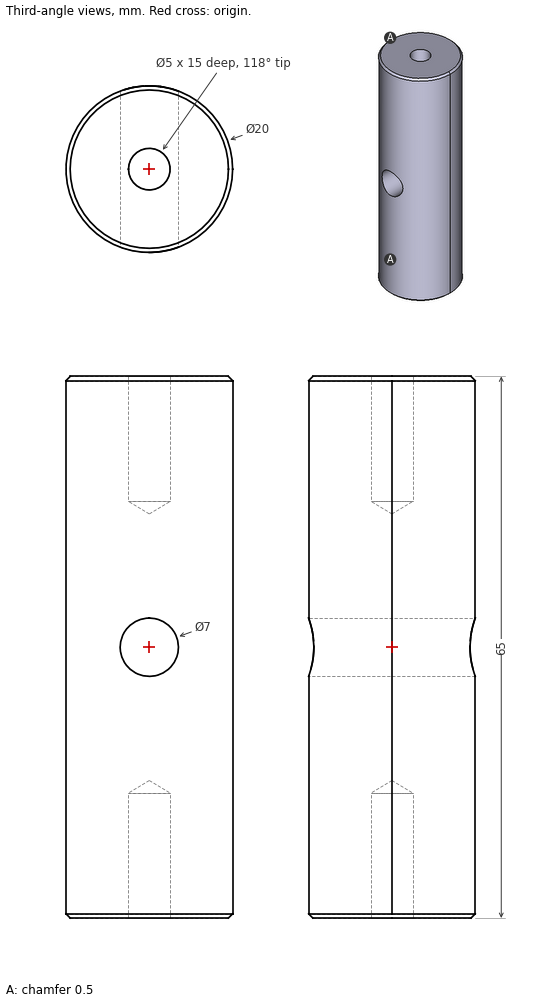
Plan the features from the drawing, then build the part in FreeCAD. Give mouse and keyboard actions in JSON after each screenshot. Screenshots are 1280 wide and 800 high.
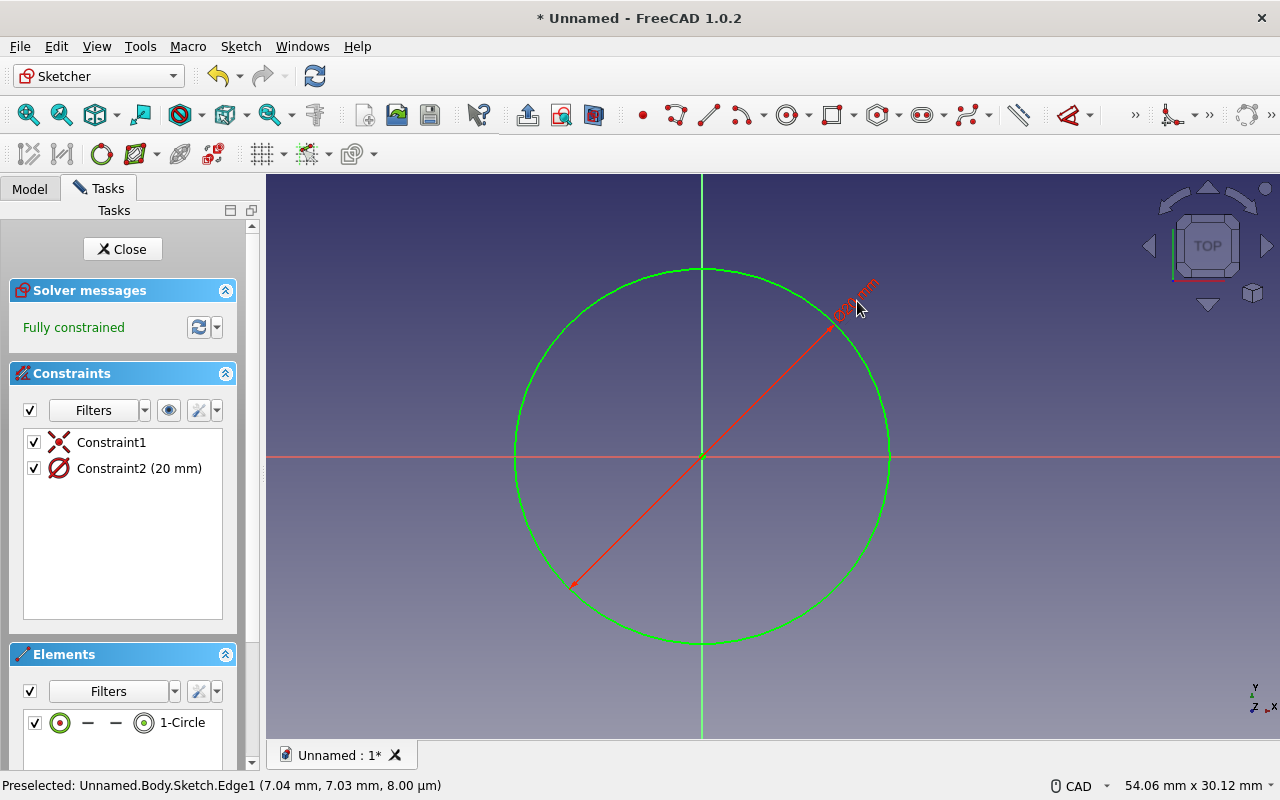
{"action": "left_click", "coordinate": [123, 249]}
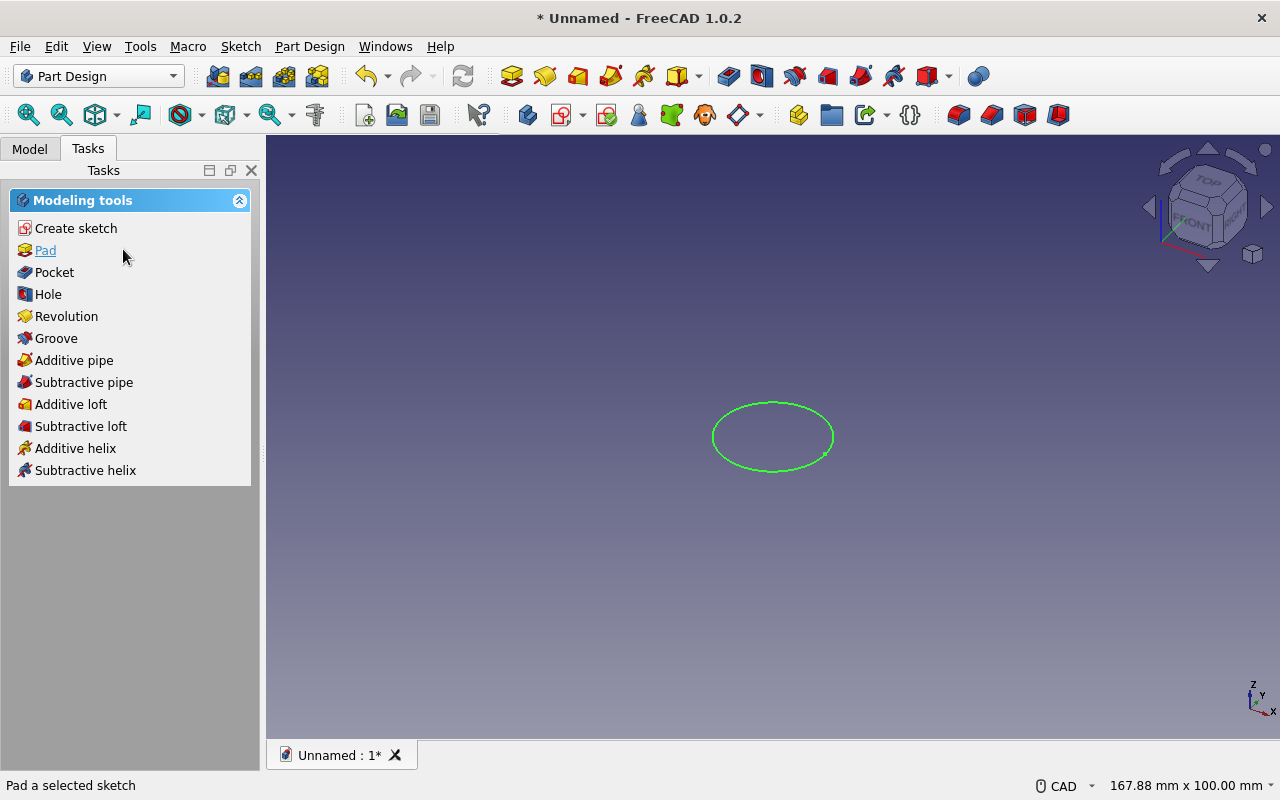
{"action": "left_click", "coordinate": [512, 76]}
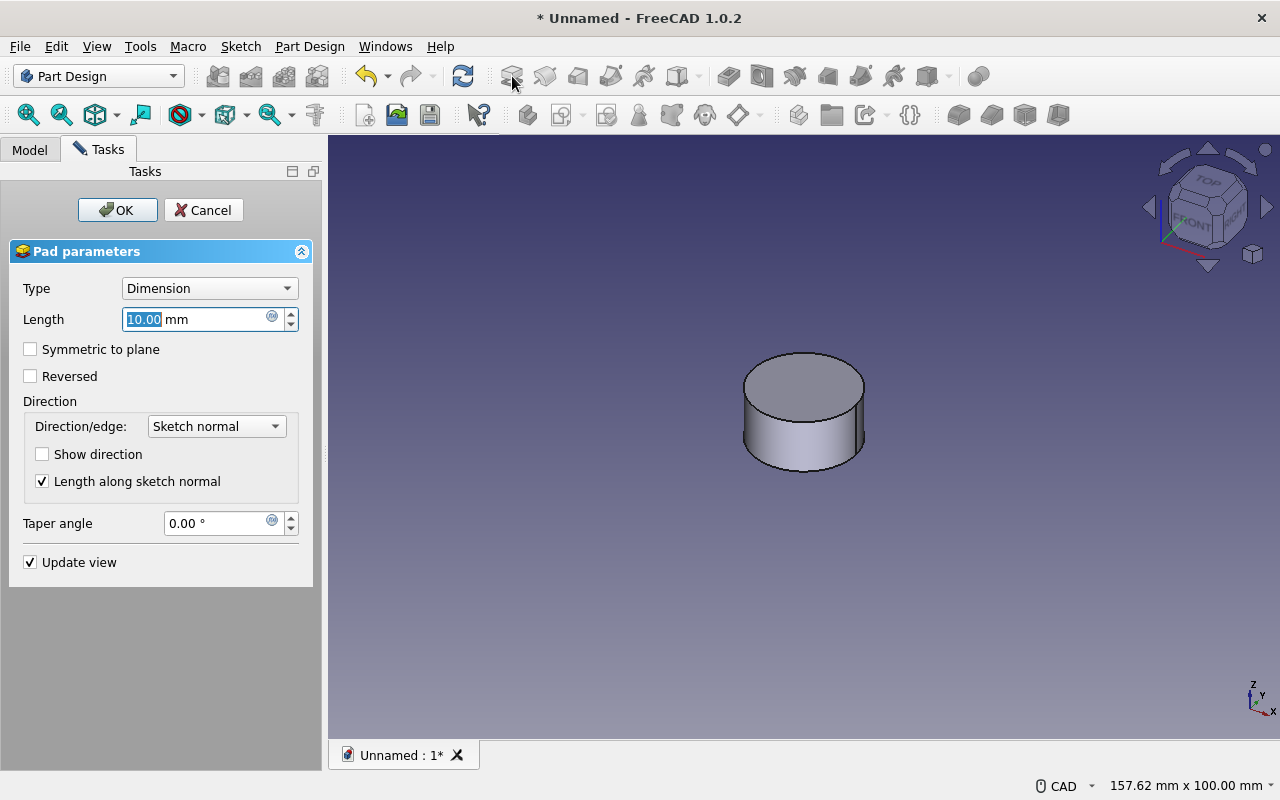
{"action": "type", "text": "65"}
{"action": "key", "text": "Tab"}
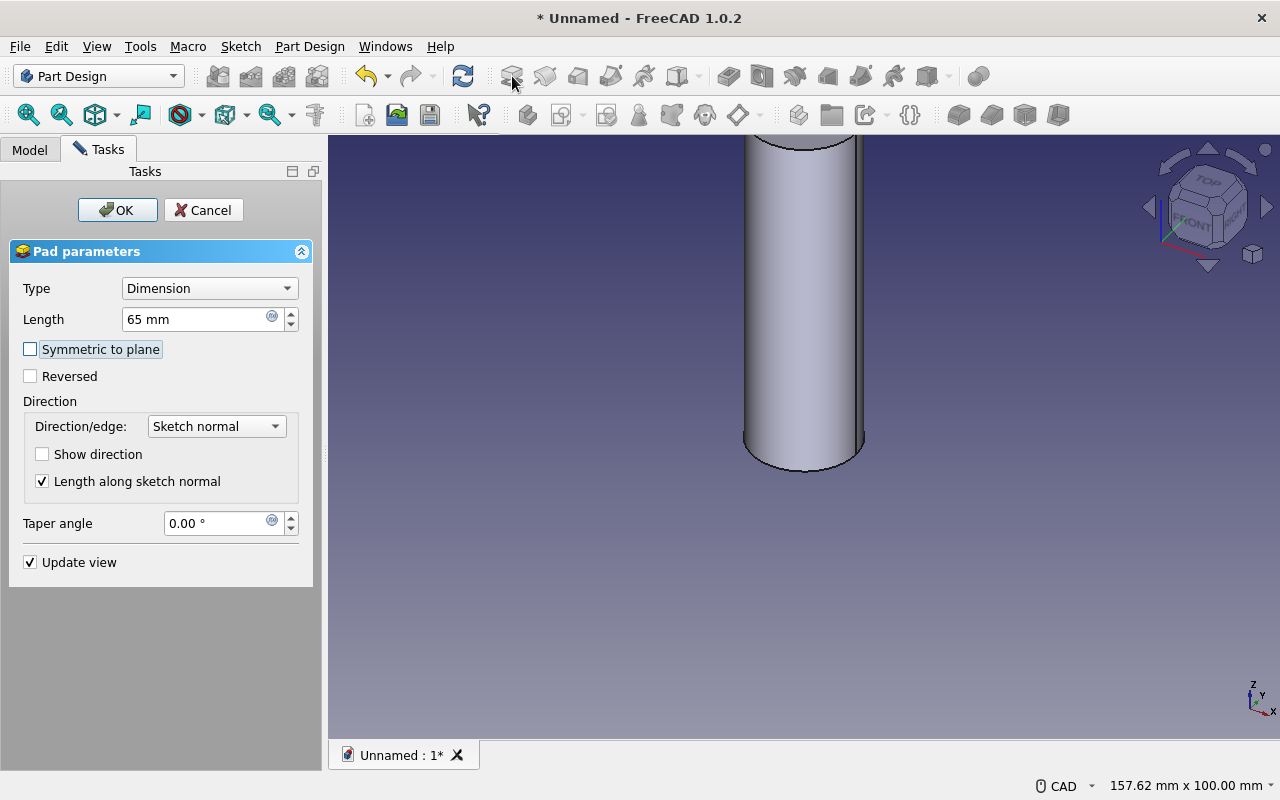
{"action": "left_click", "coordinate": [31, 349]}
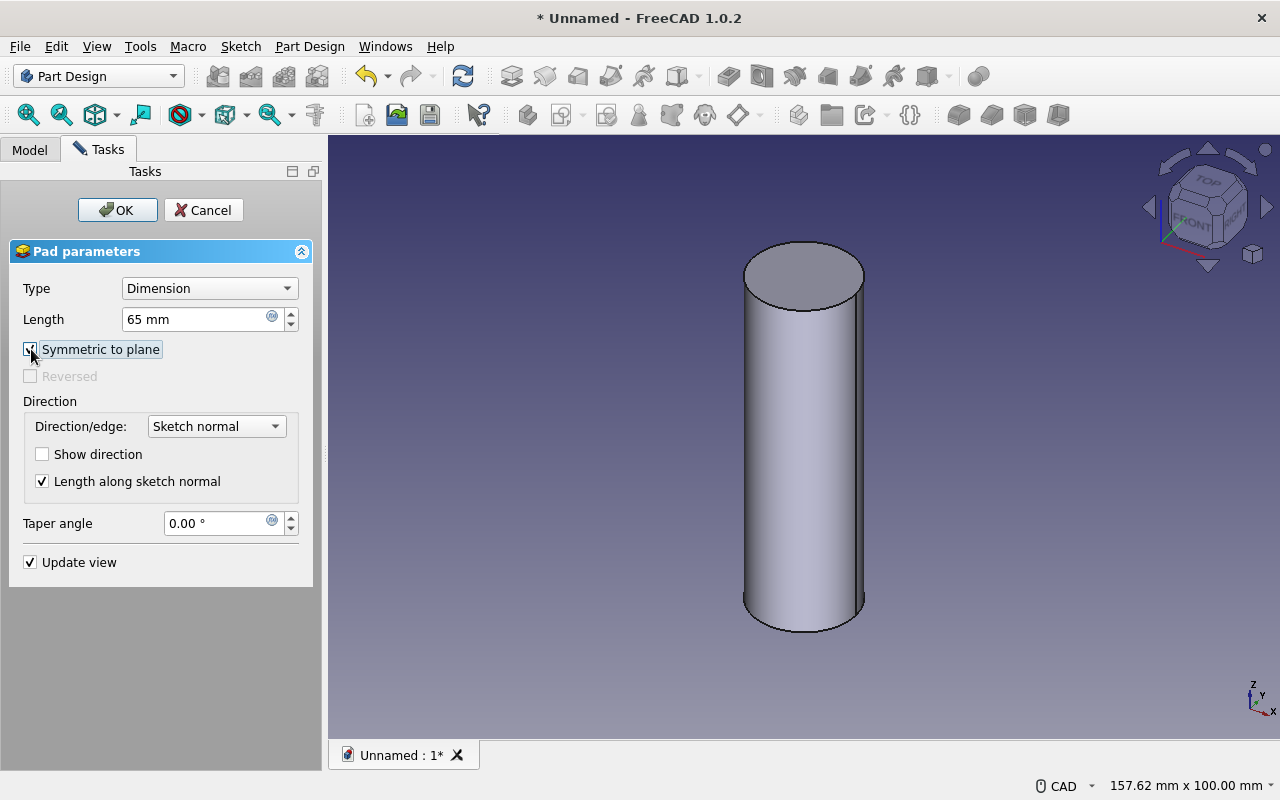
{"action": "left_click", "coordinate": [118, 210]}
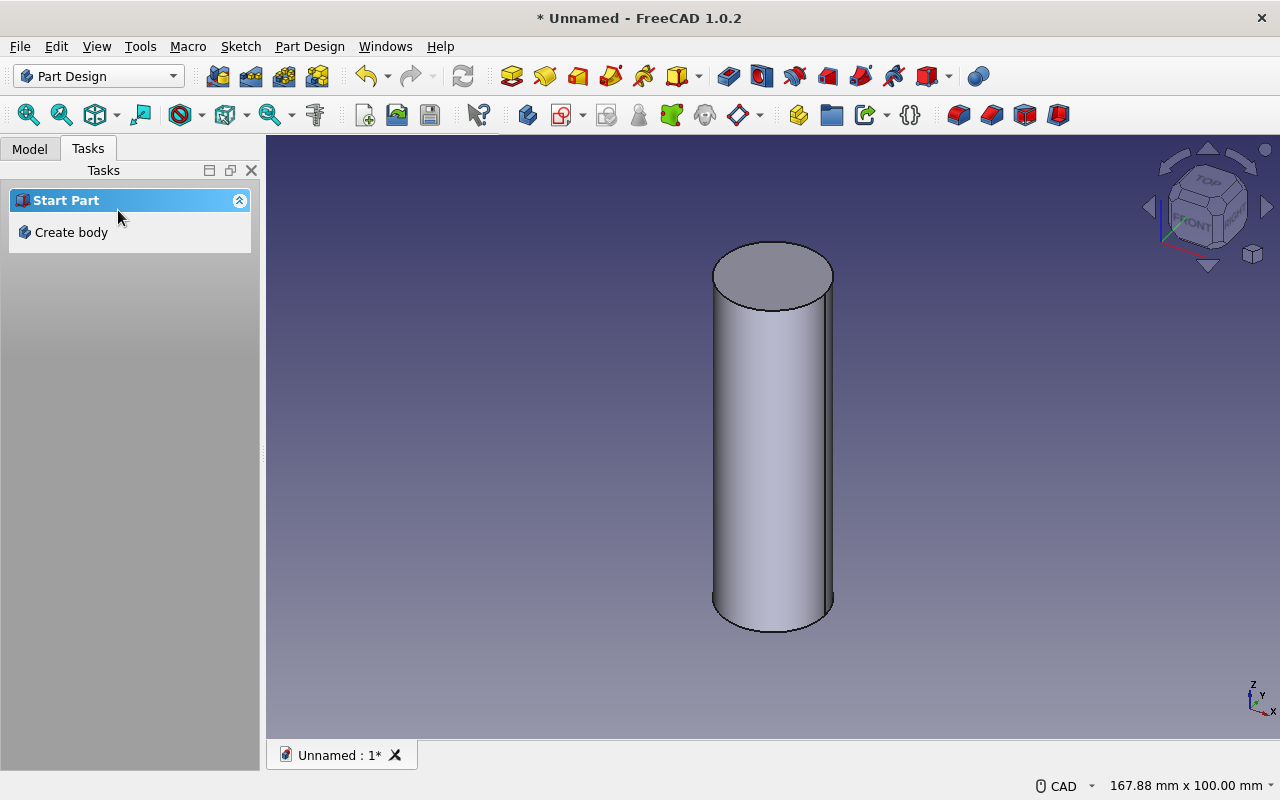
{"action": "left_click", "coordinate": [713, 279]}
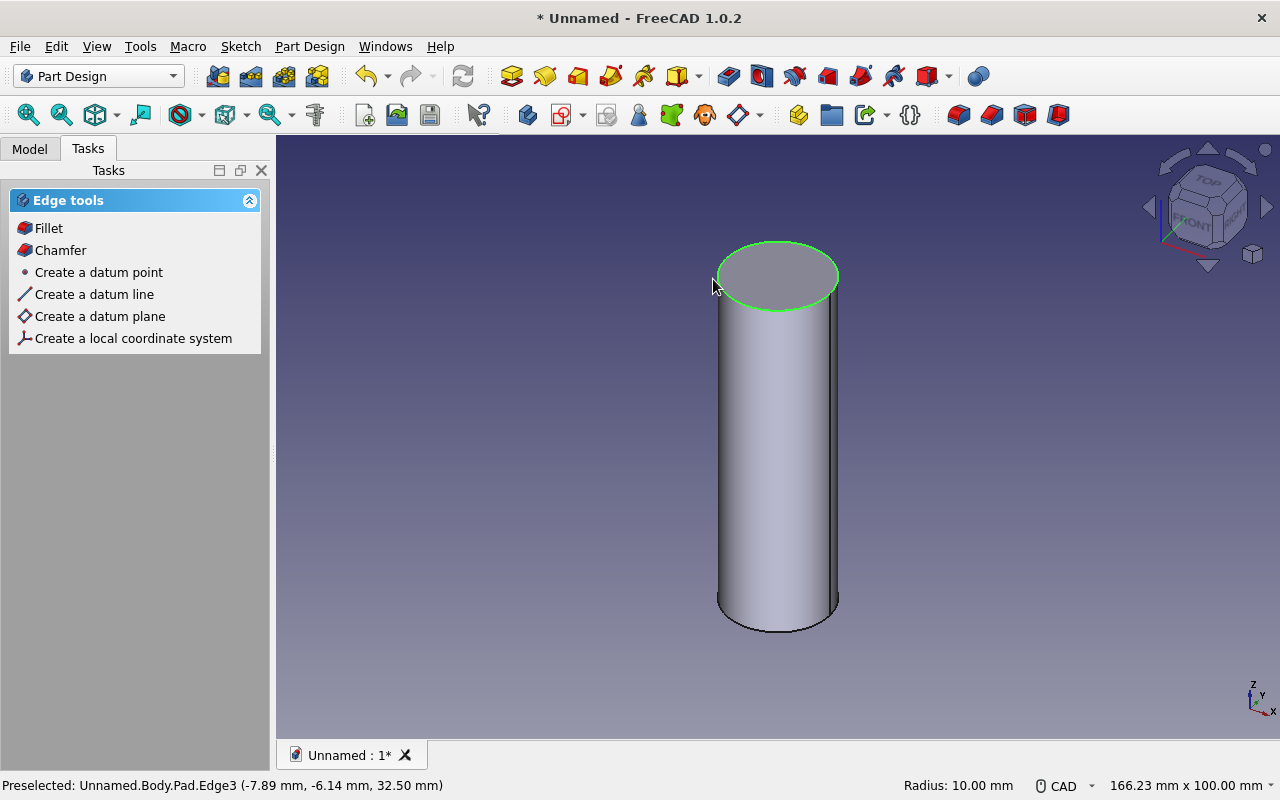
{"action": "key", "text": "0"}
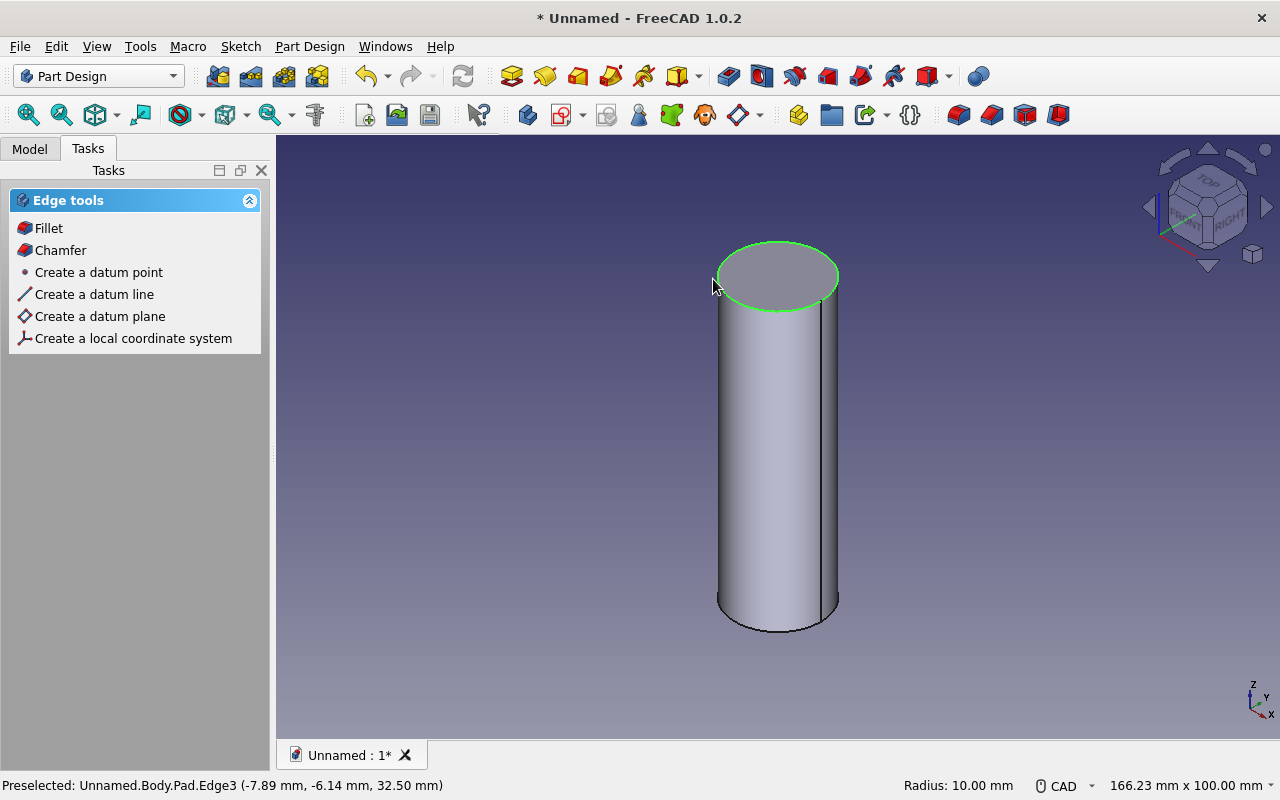
{"action": "left_click", "coordinate": [724, 612], "text": "ctrl"}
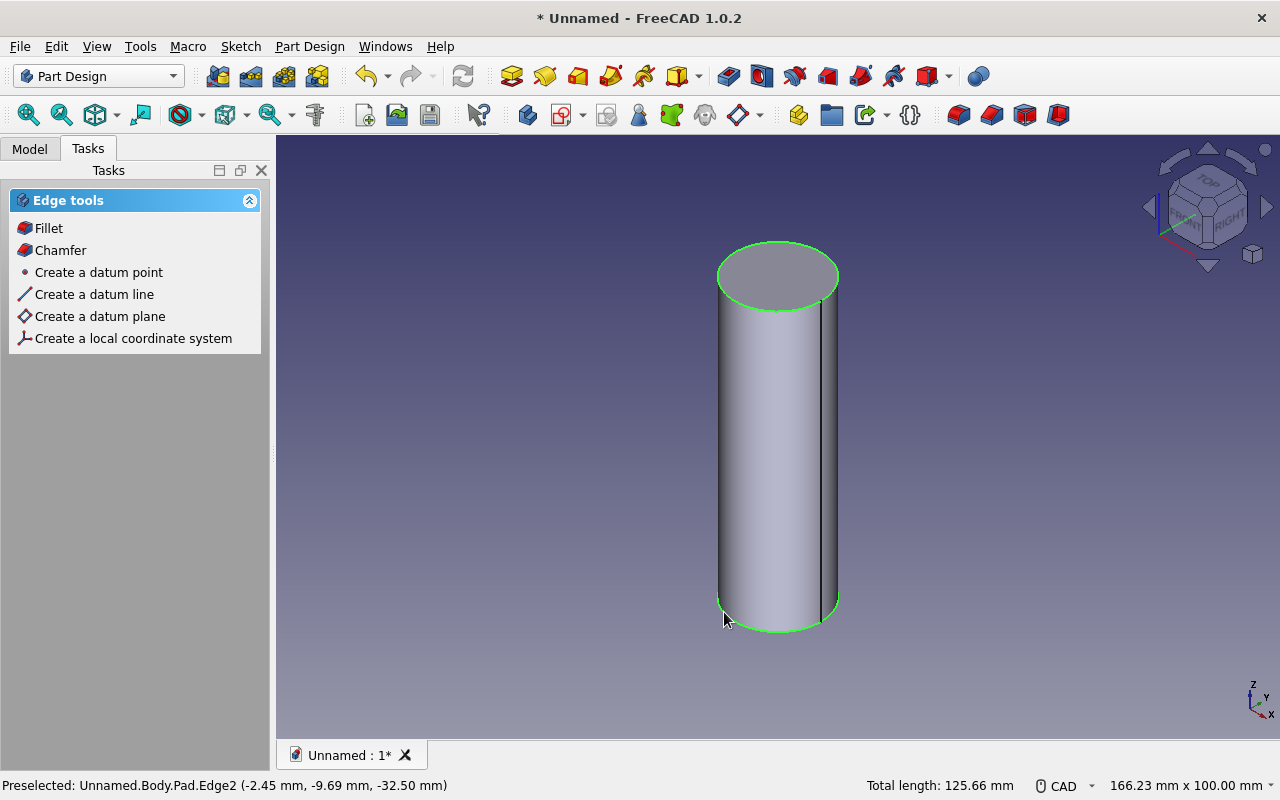
{"action": "left_click", "coordinate": [992, 116]}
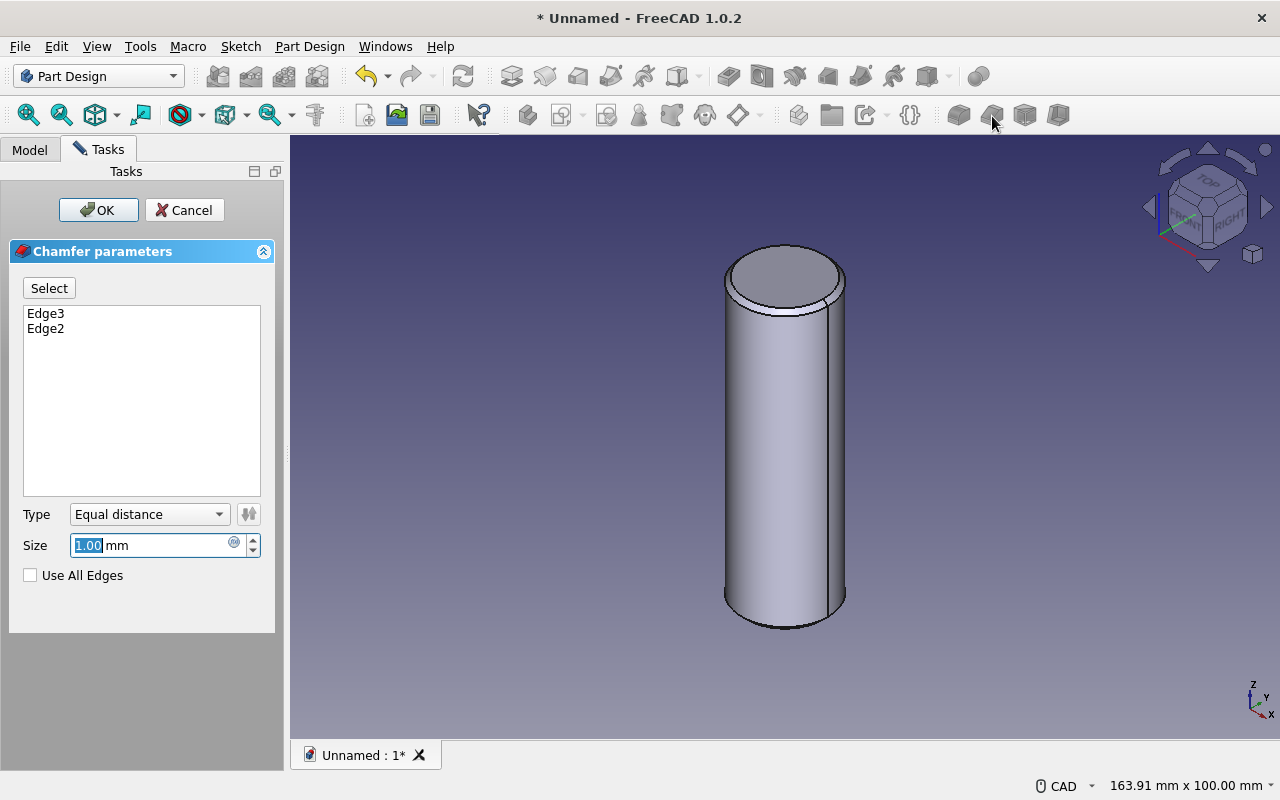
{"action": "type", "text": "0.5"}
{"action": "key", "text": "Tab"}